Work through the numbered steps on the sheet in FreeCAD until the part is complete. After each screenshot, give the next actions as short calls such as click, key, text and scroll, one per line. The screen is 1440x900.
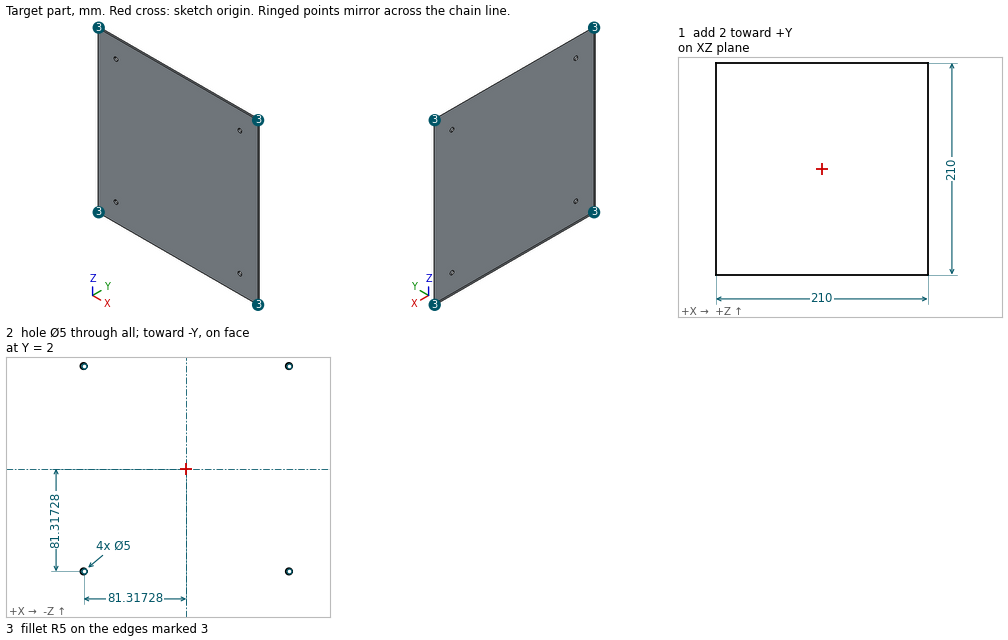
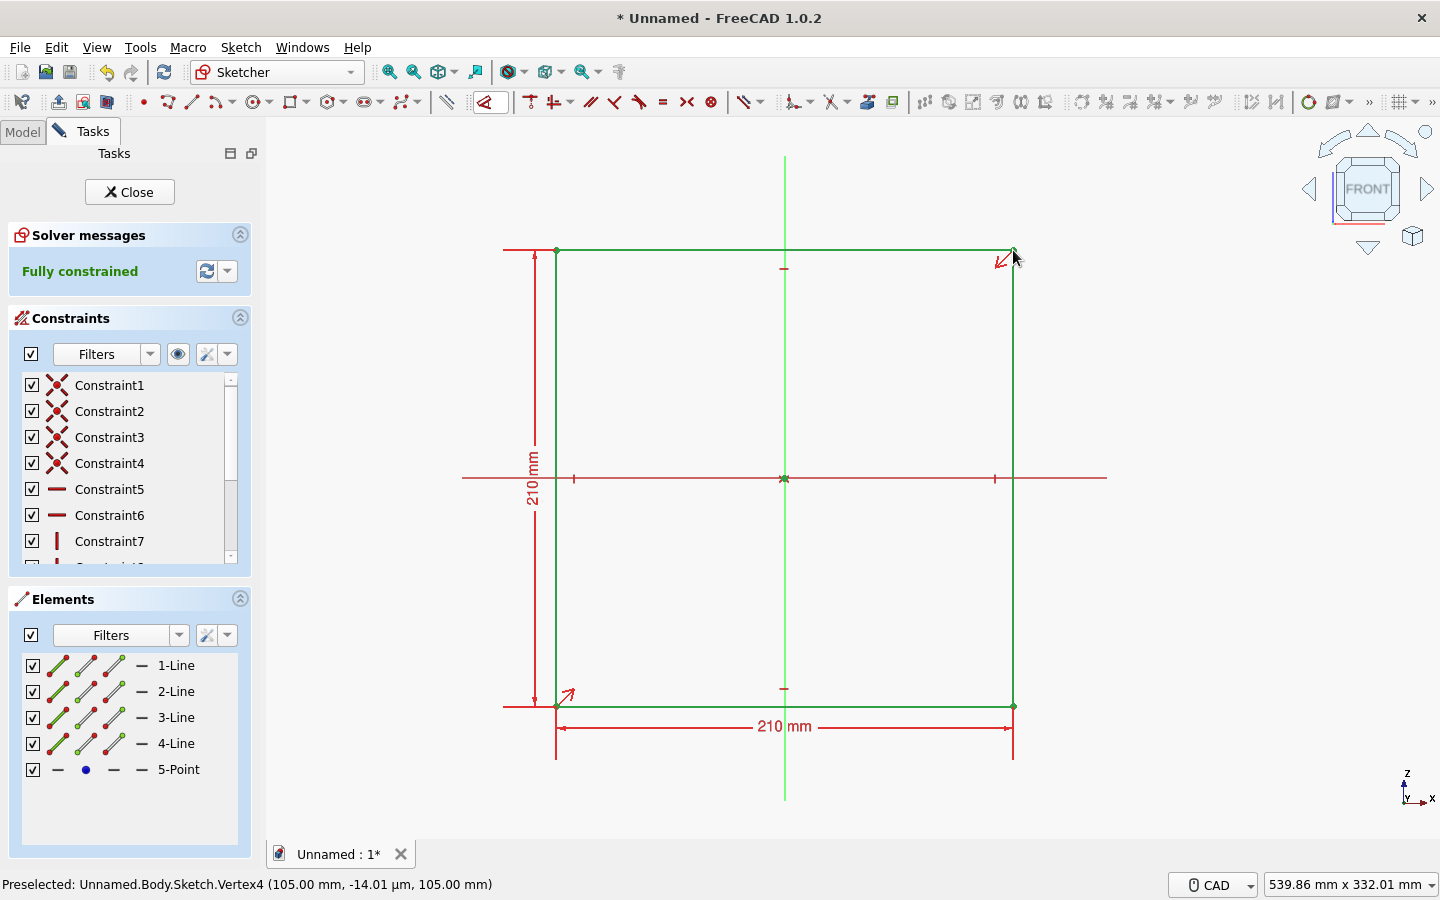
click(130, 192)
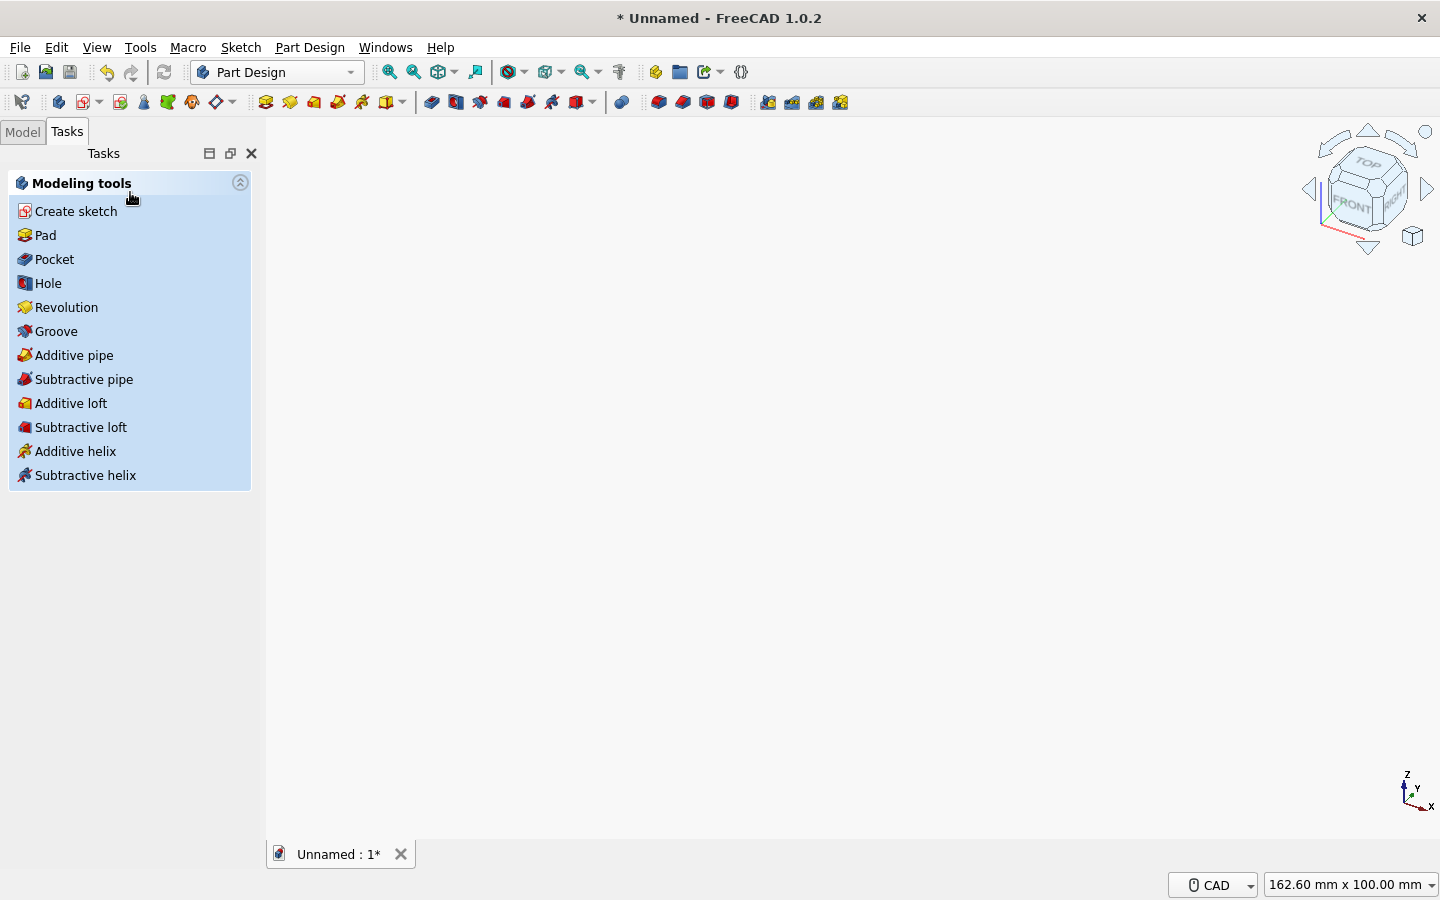
click(266, 102)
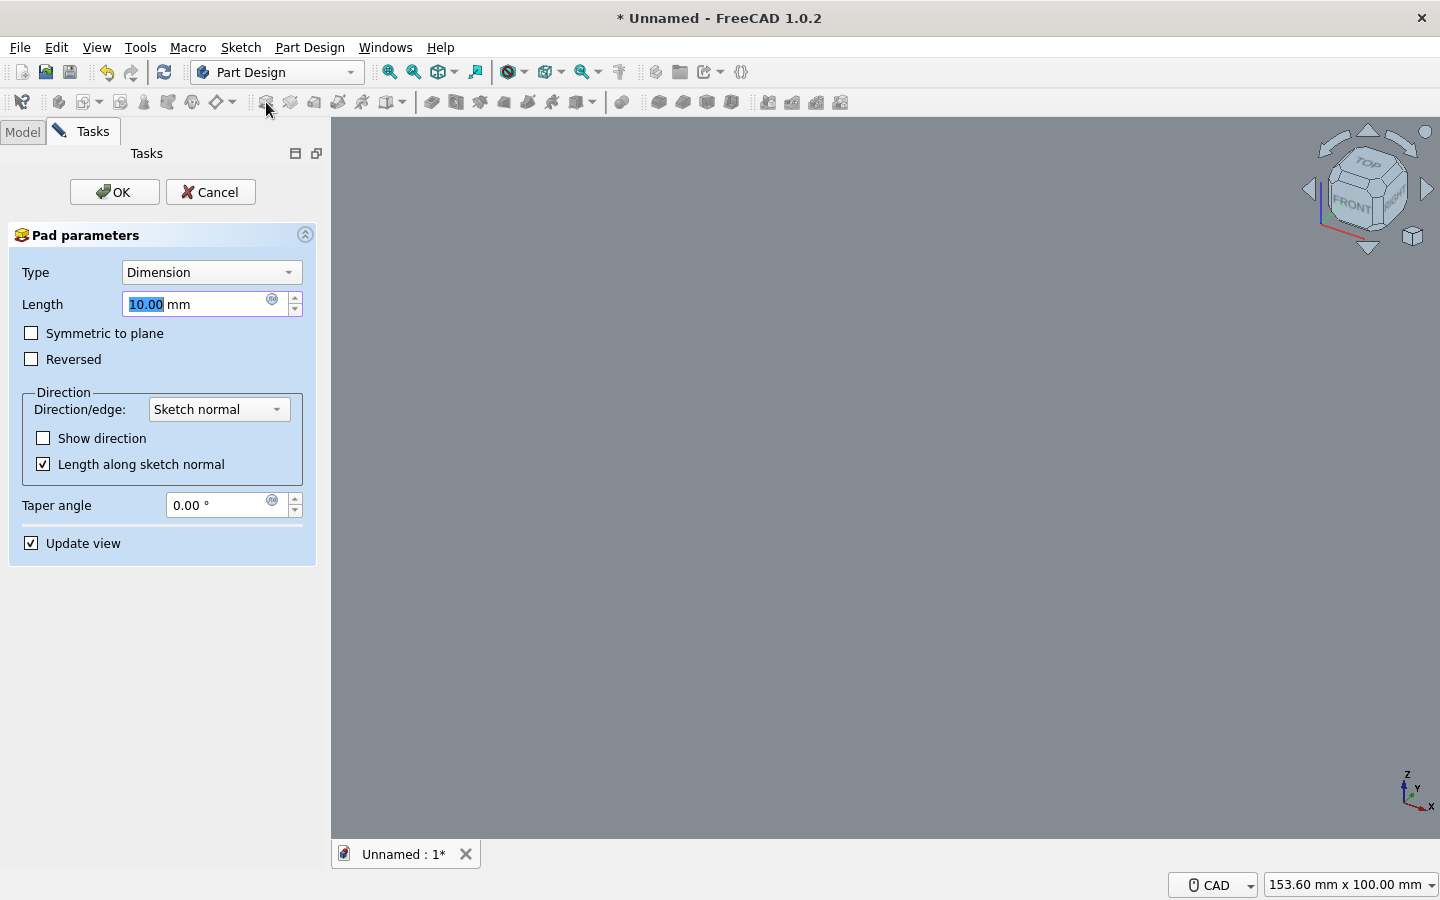
text(2)
key(Tab)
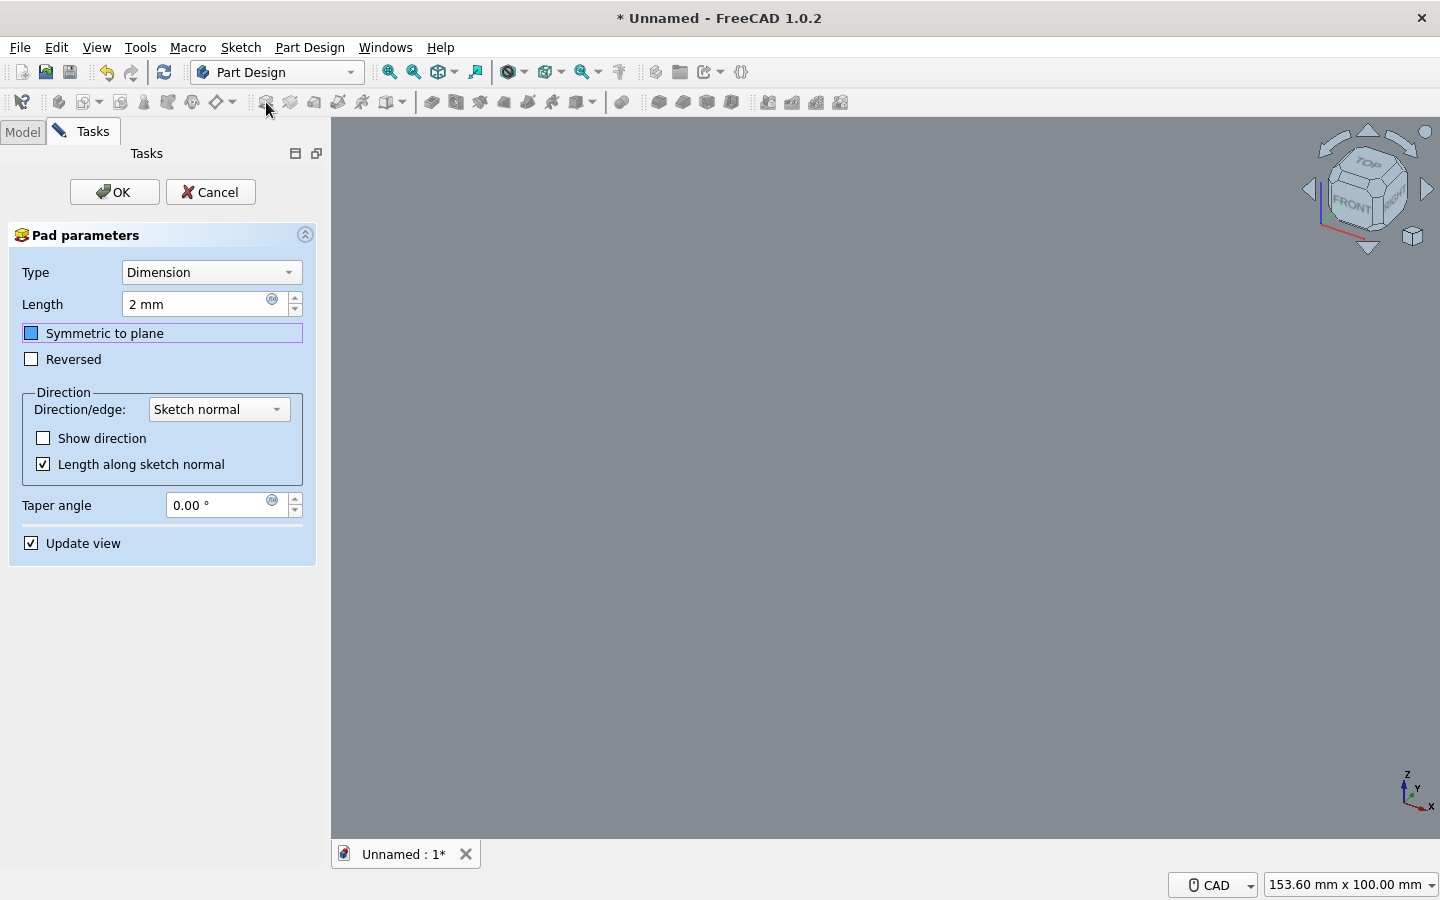
click(30, 359)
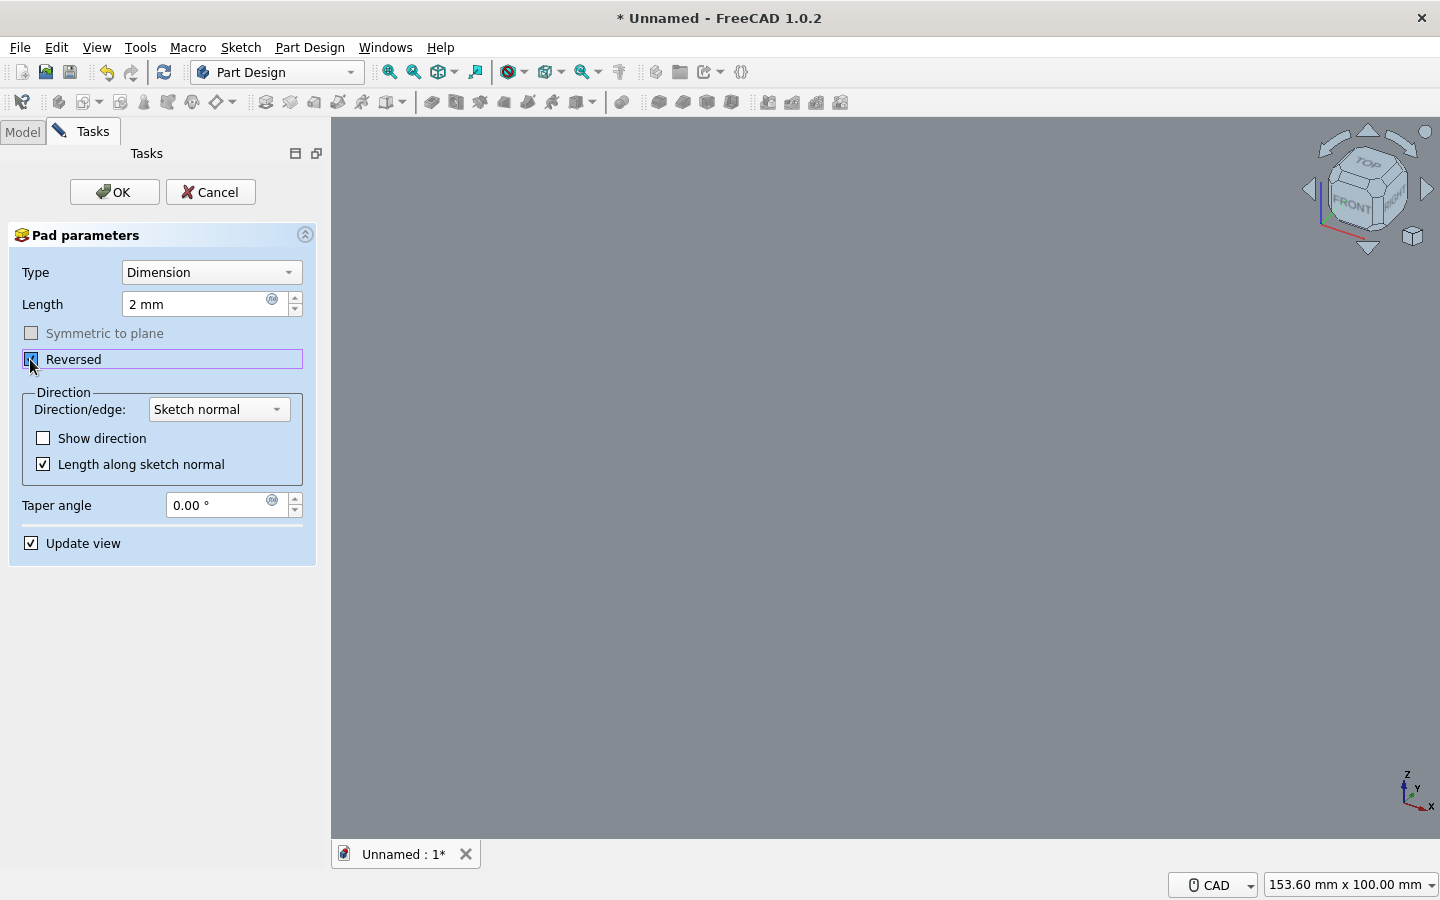
click(115, 192)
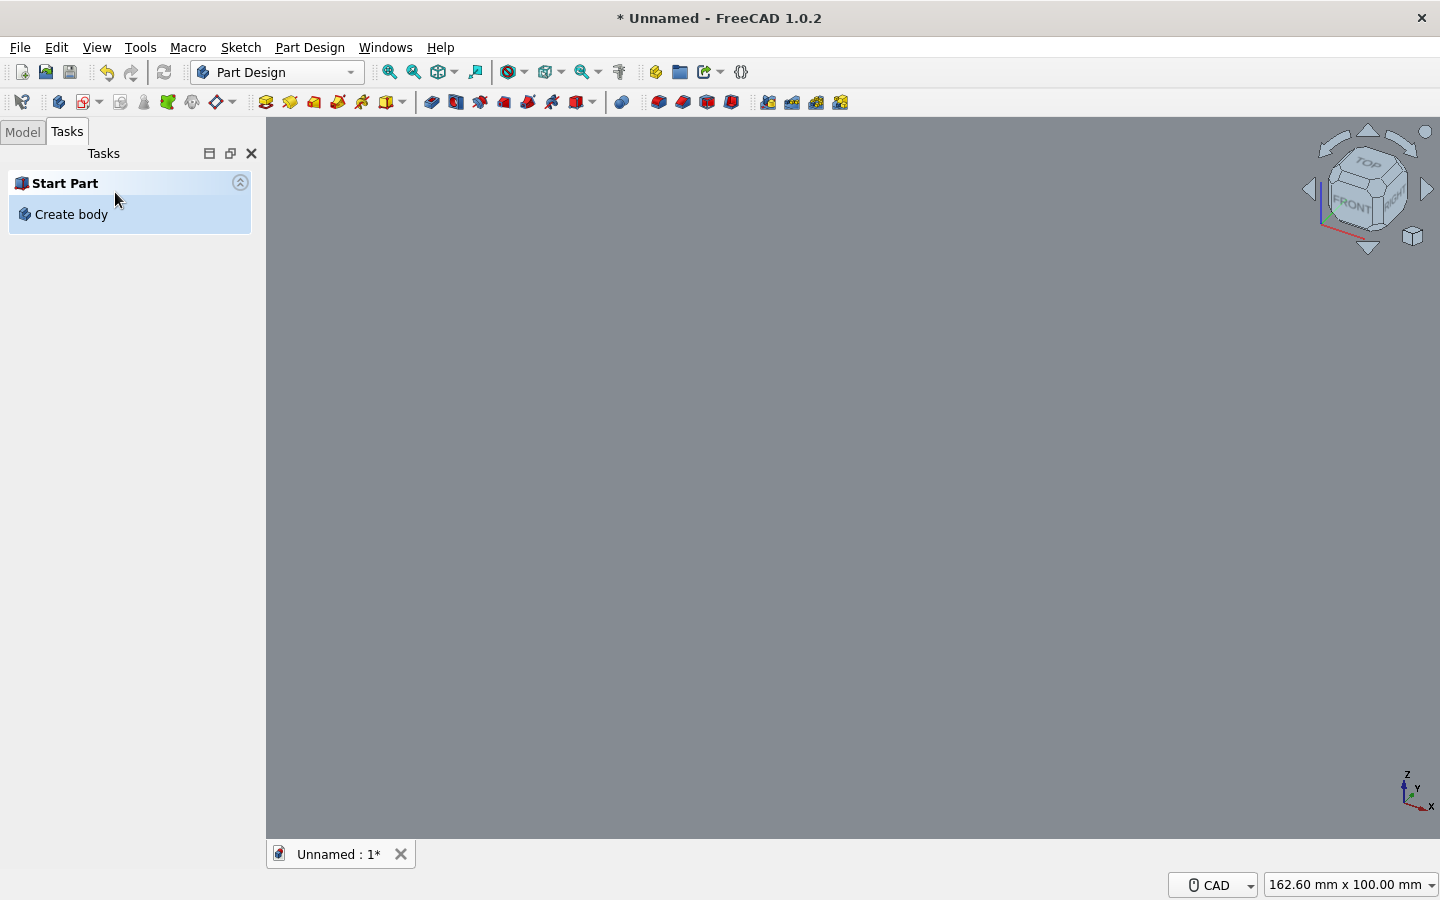
click(390, 72)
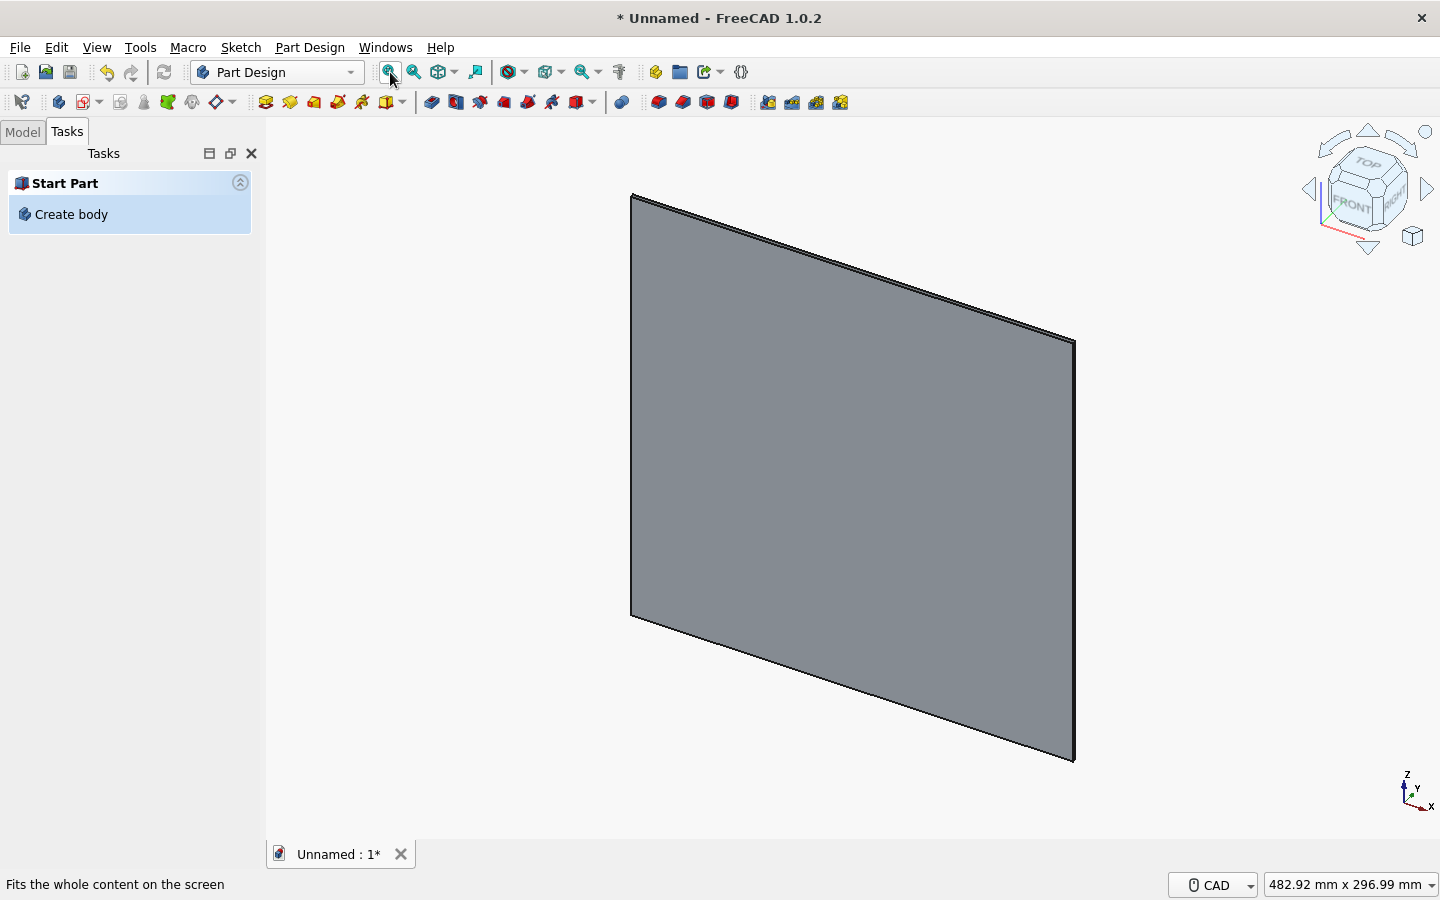
key(4)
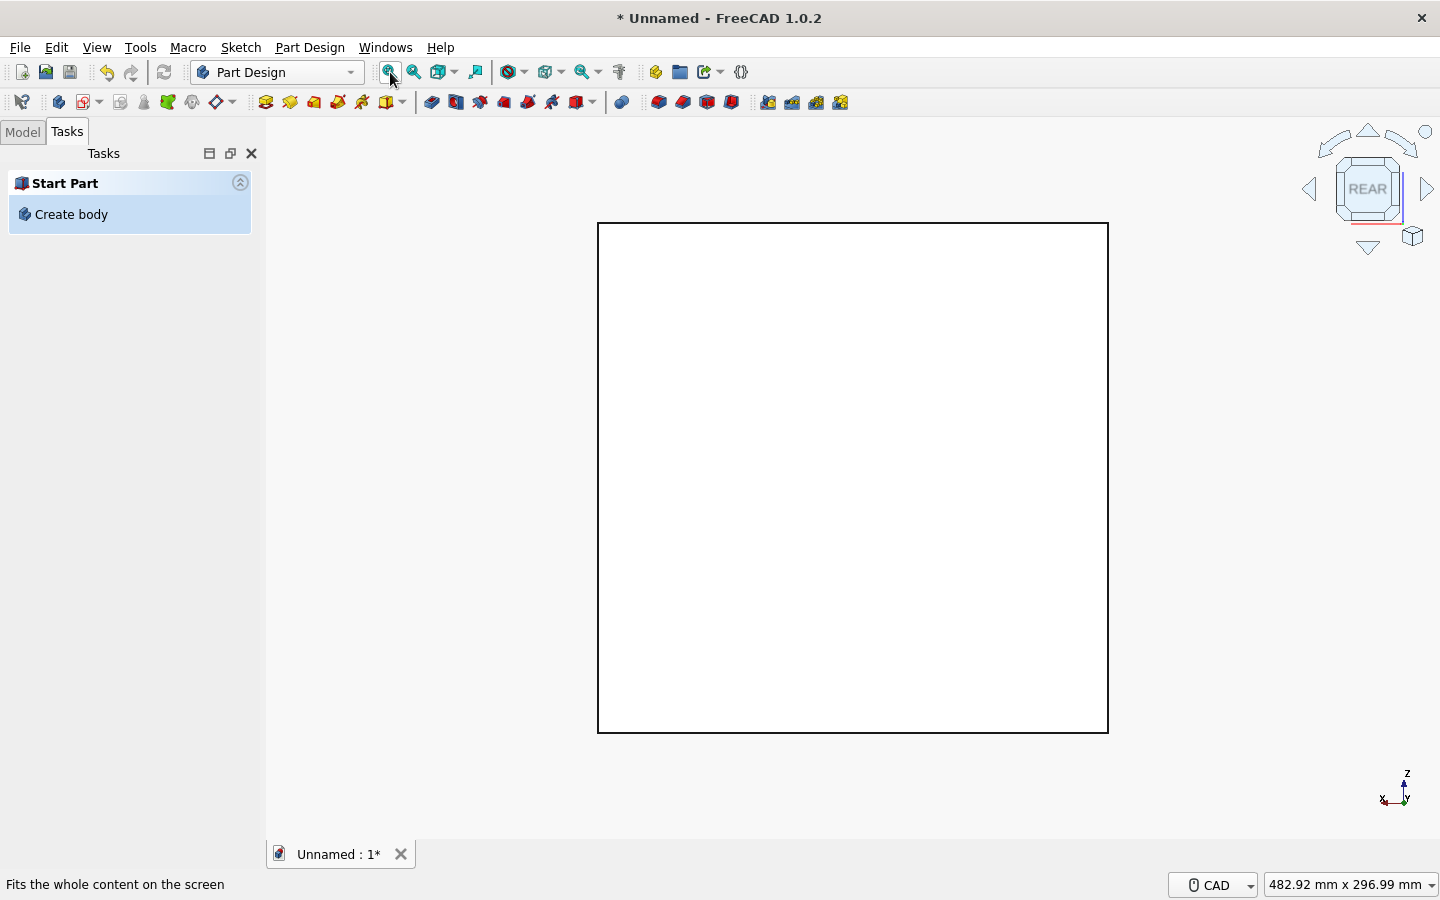
click(853, 477)